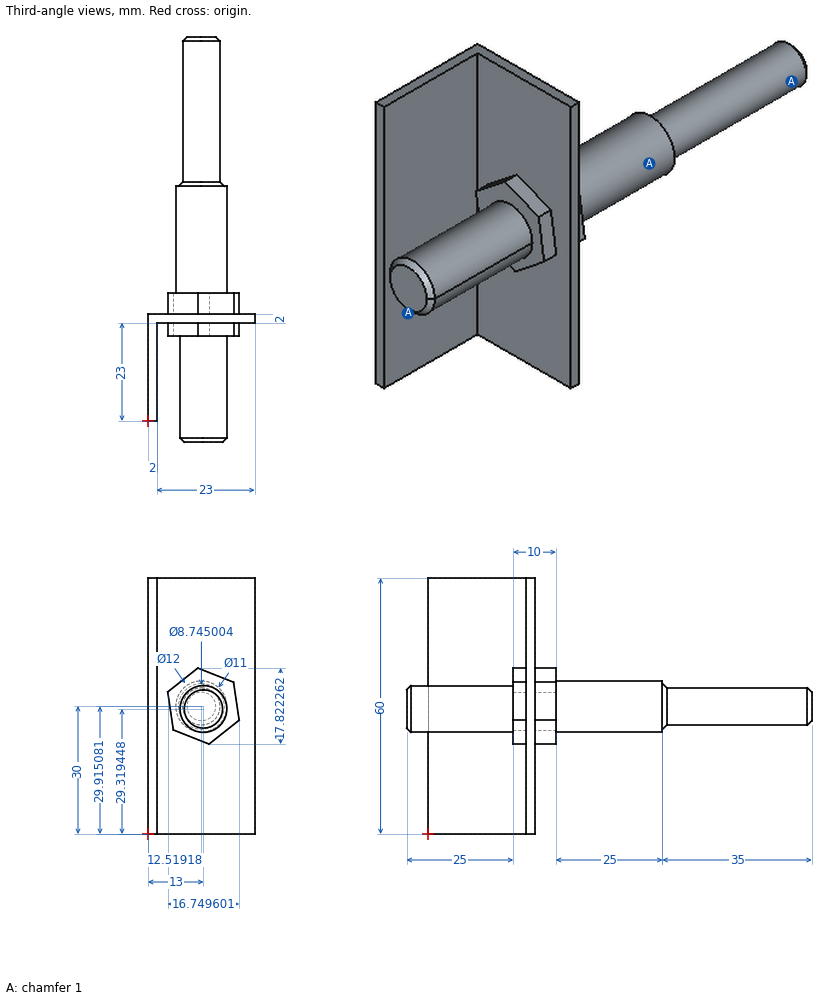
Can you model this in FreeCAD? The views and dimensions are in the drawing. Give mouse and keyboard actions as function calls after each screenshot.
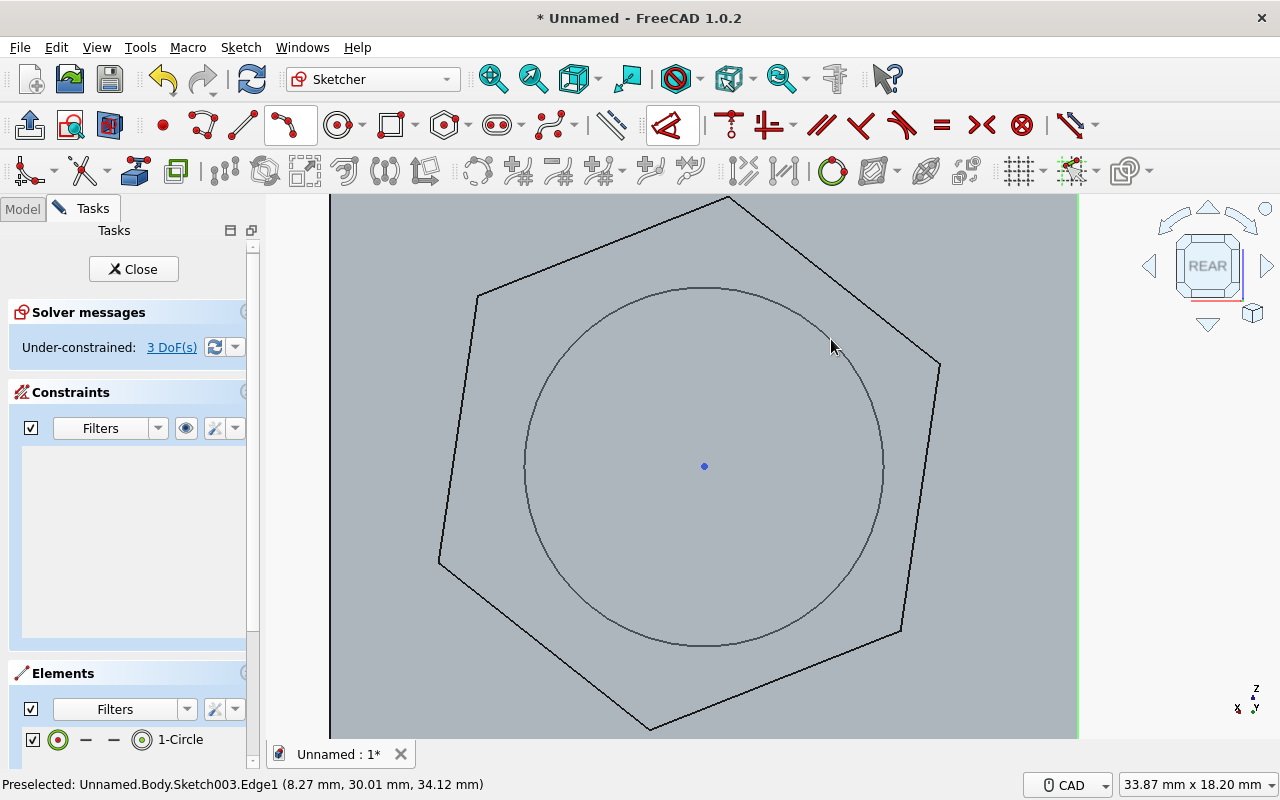
click(831, 340)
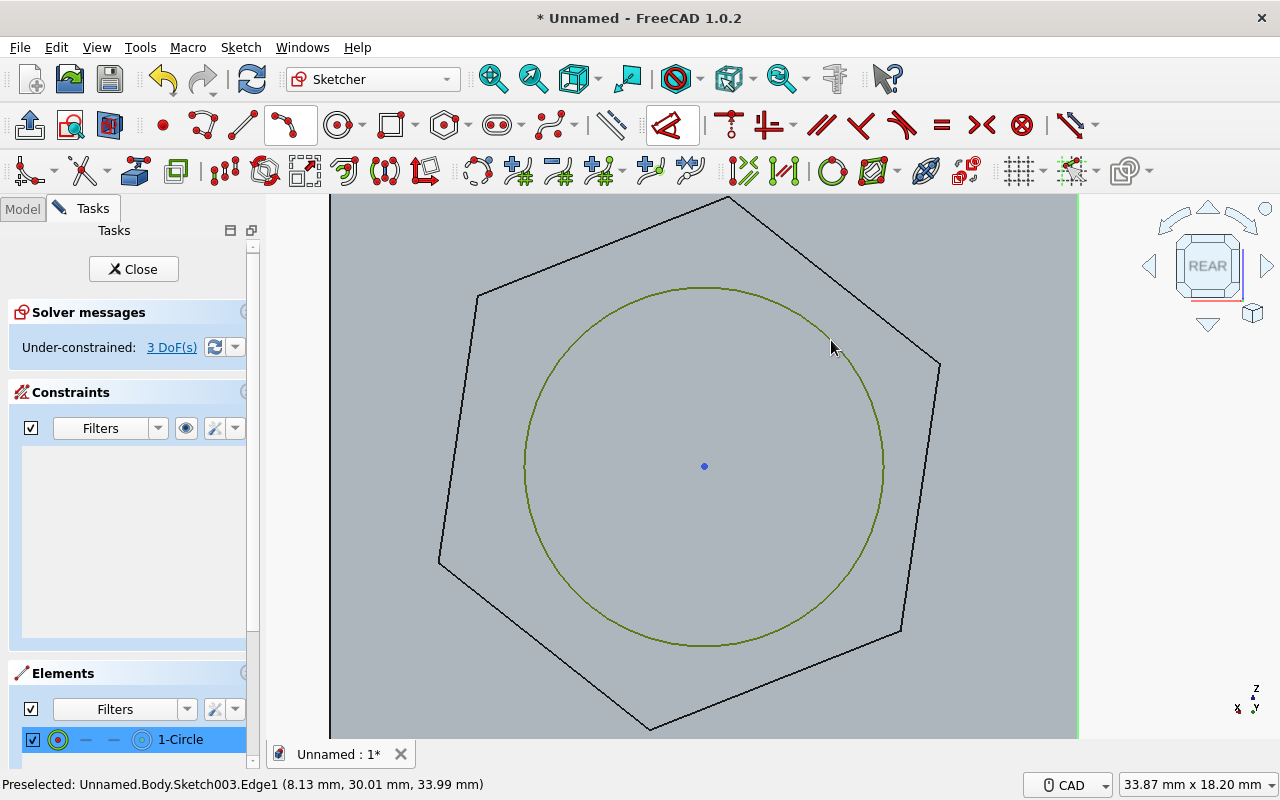
key(k)
key(o)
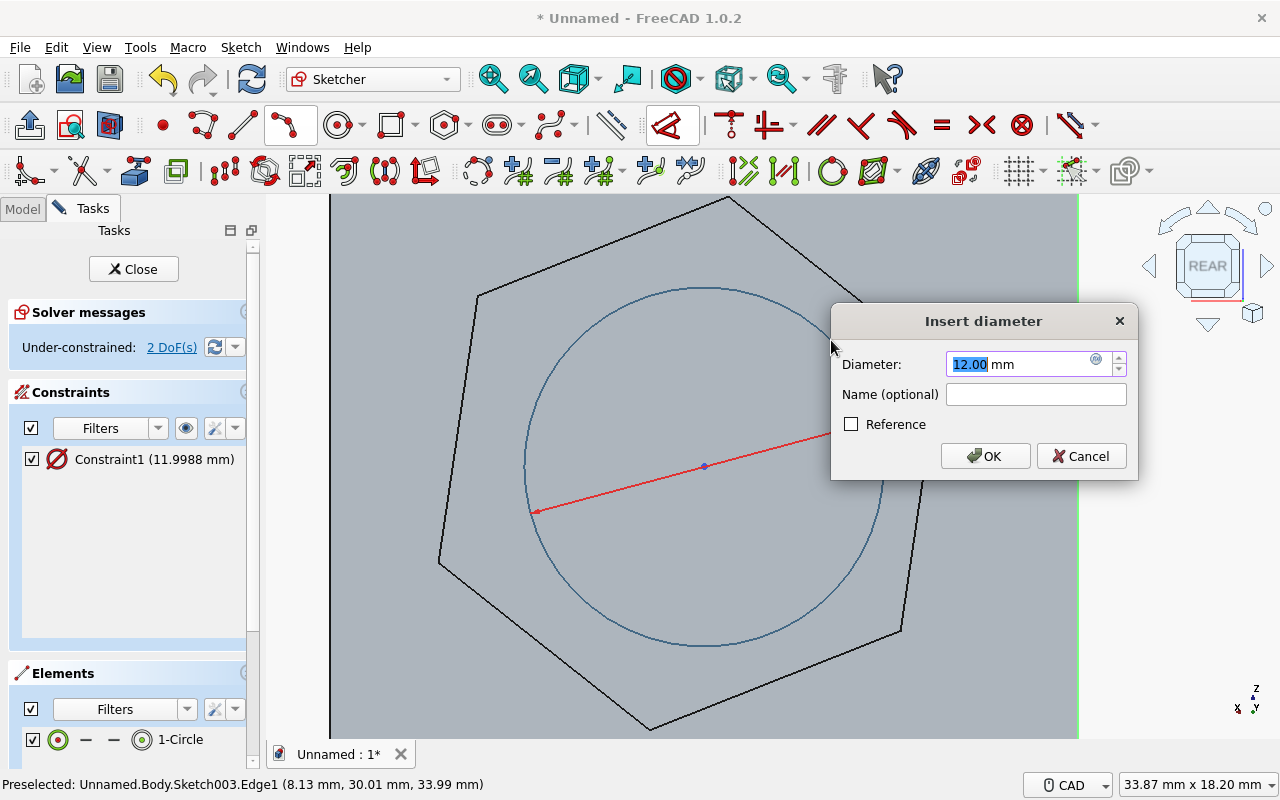
text(12)
key(Return)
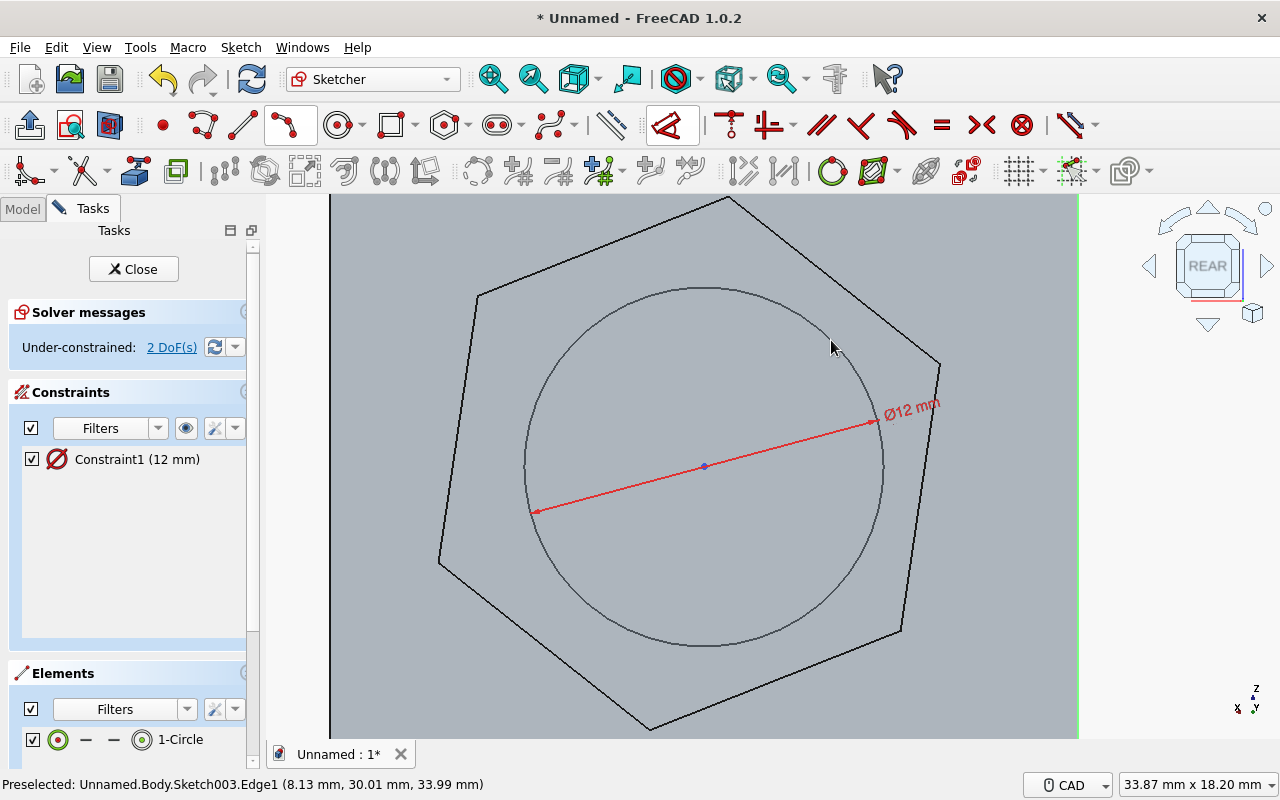
click(704, 467)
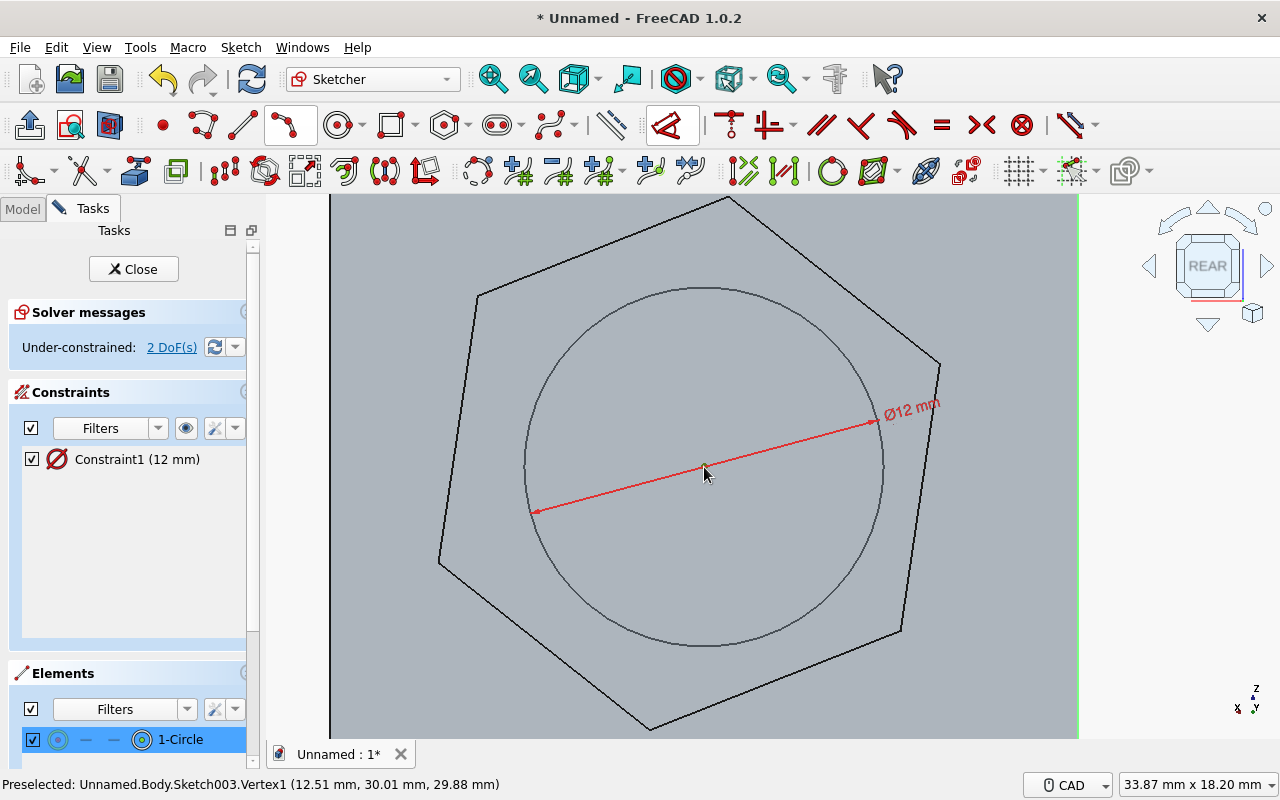
click(694, 126)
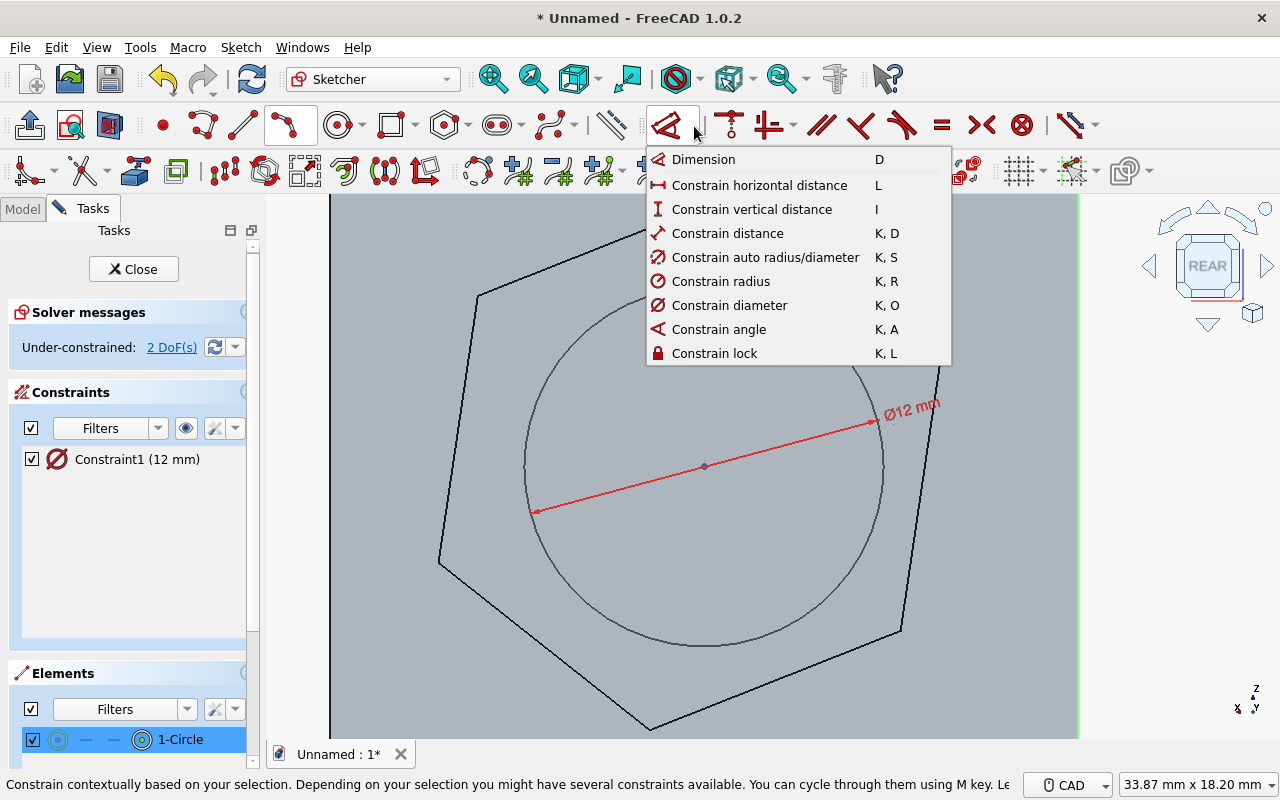
click(799, 185)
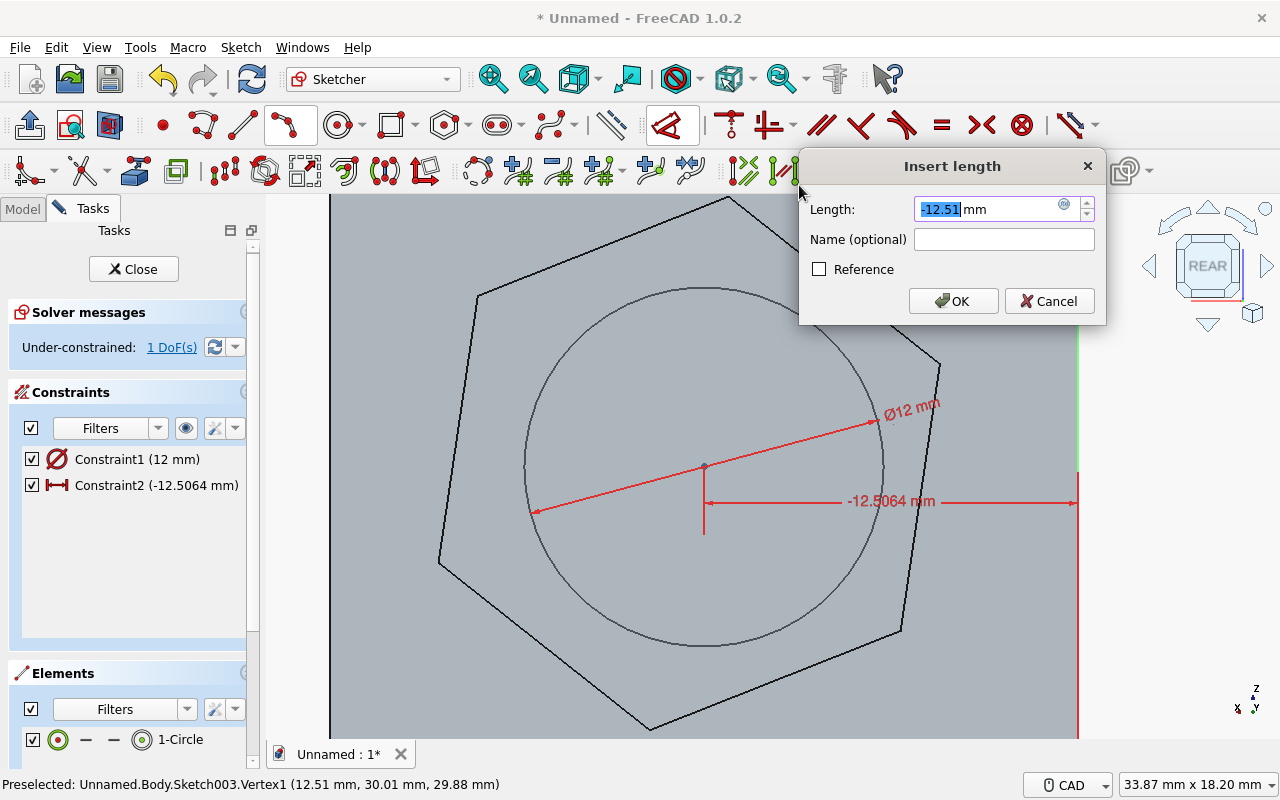
text(-12.51918)
key(Return)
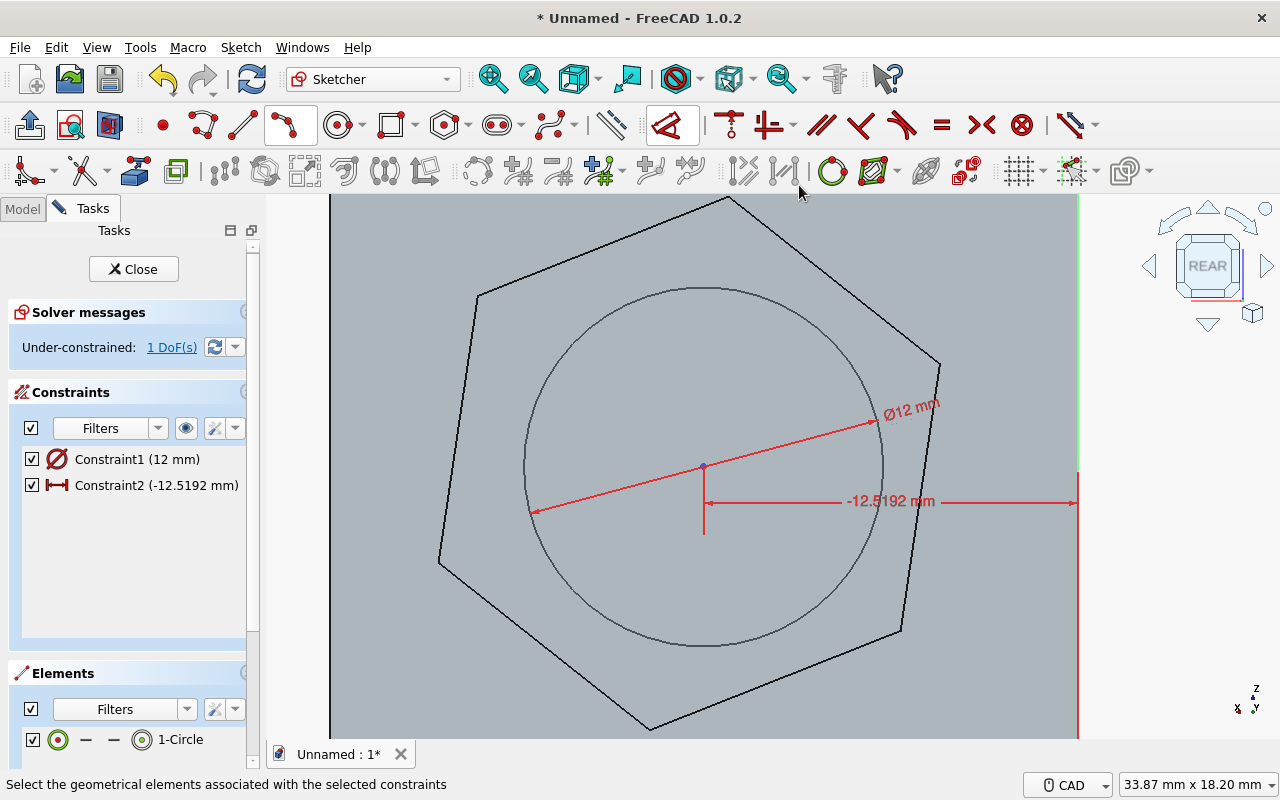
click(704, 467)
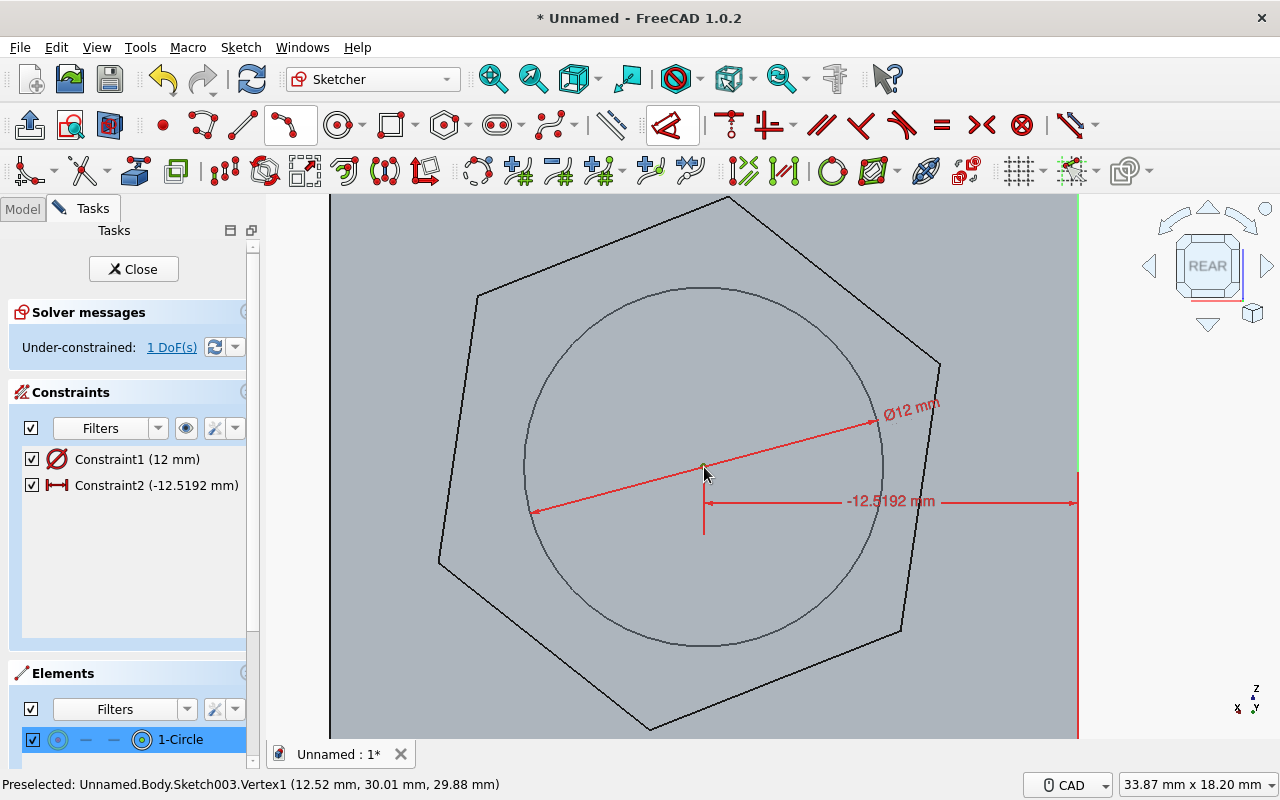
click(694, 126)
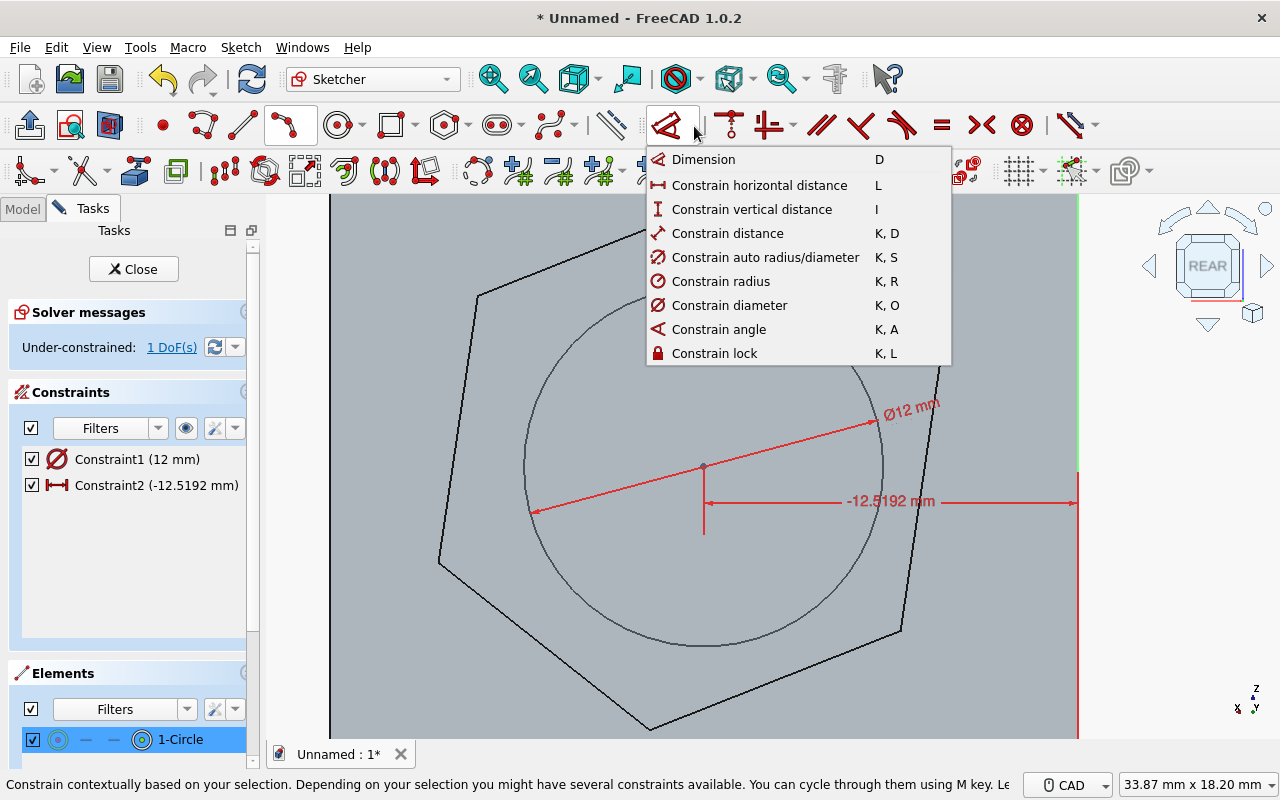
click(799, 209)